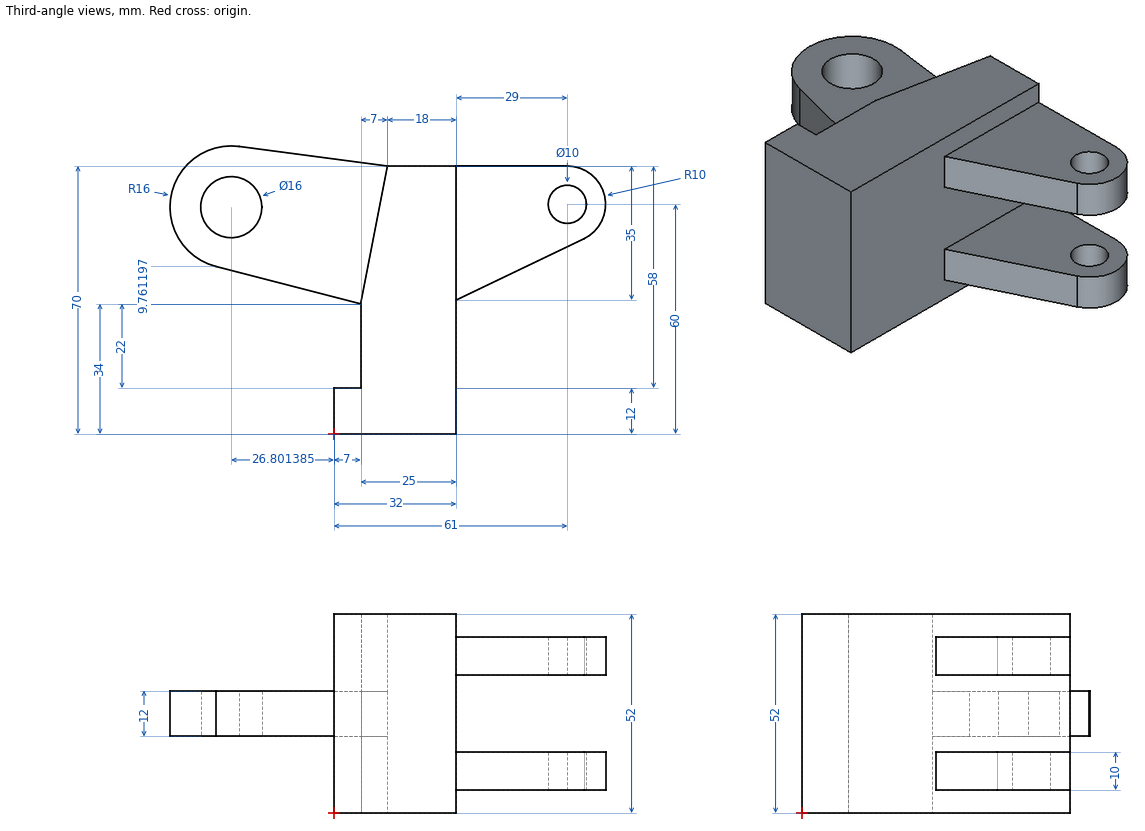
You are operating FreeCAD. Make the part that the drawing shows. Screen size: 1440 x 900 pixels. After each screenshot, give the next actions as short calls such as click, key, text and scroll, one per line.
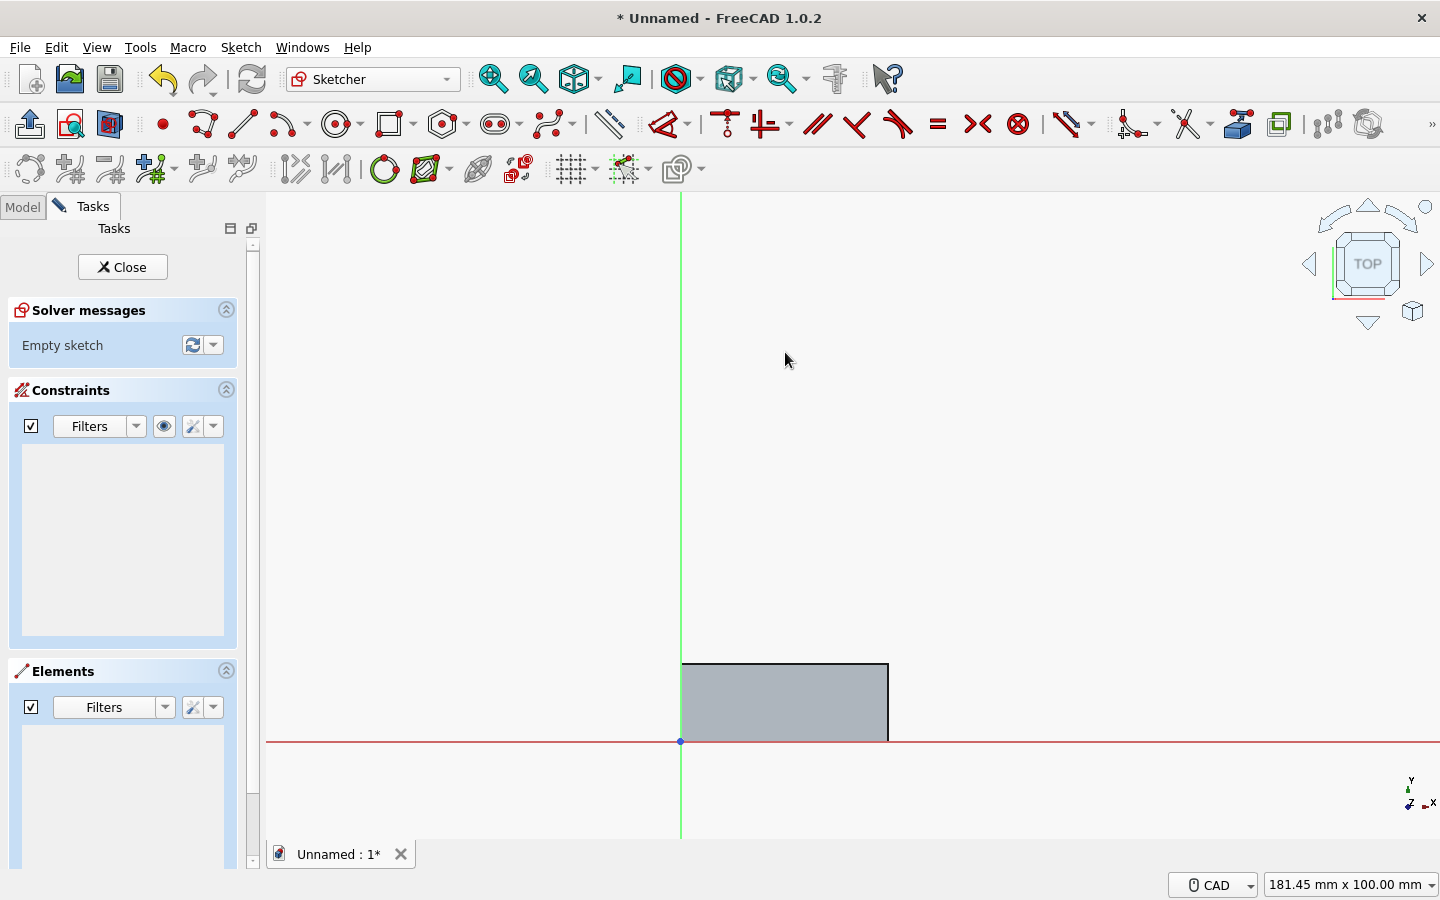
key(g)
key(m)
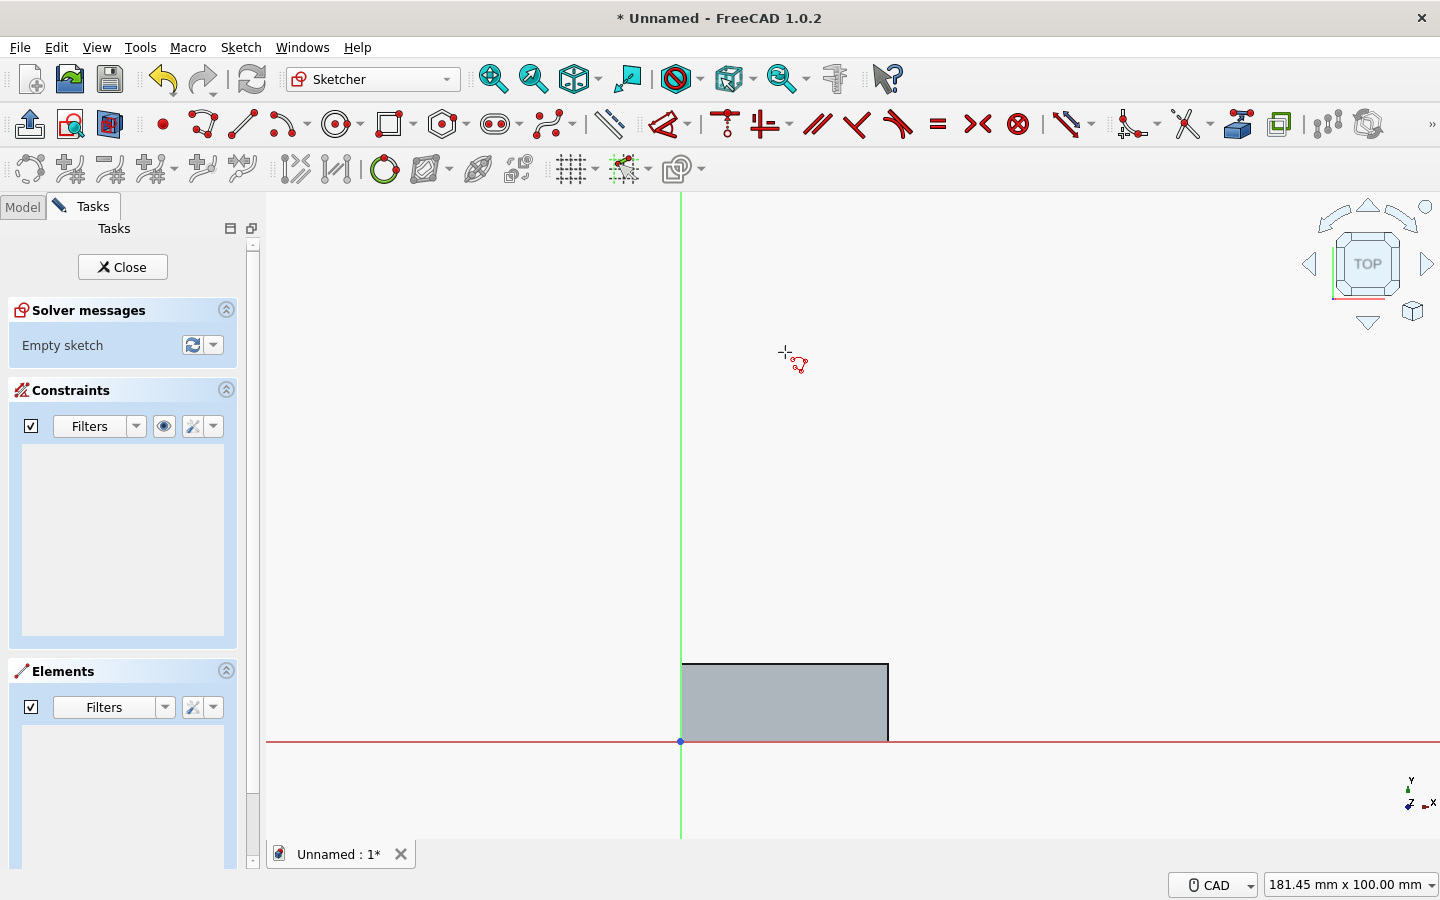
click(726, 664)
click(888, 664)
click(888, 289)
click(771, 289)
click(726, 522)
click(726, 665)
key(Escape)
key(Escape)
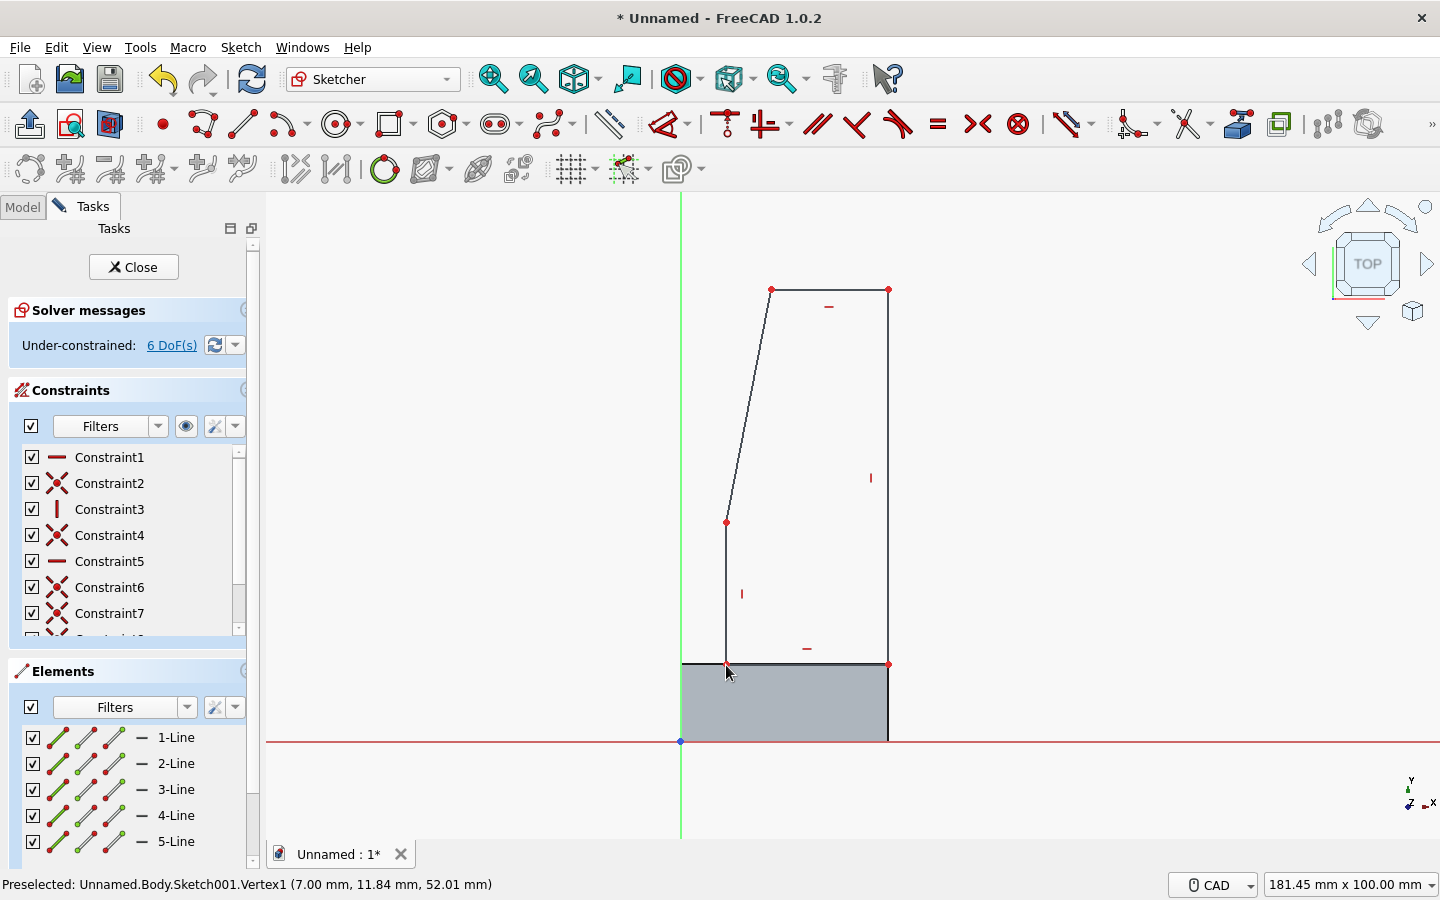
click(664, 124)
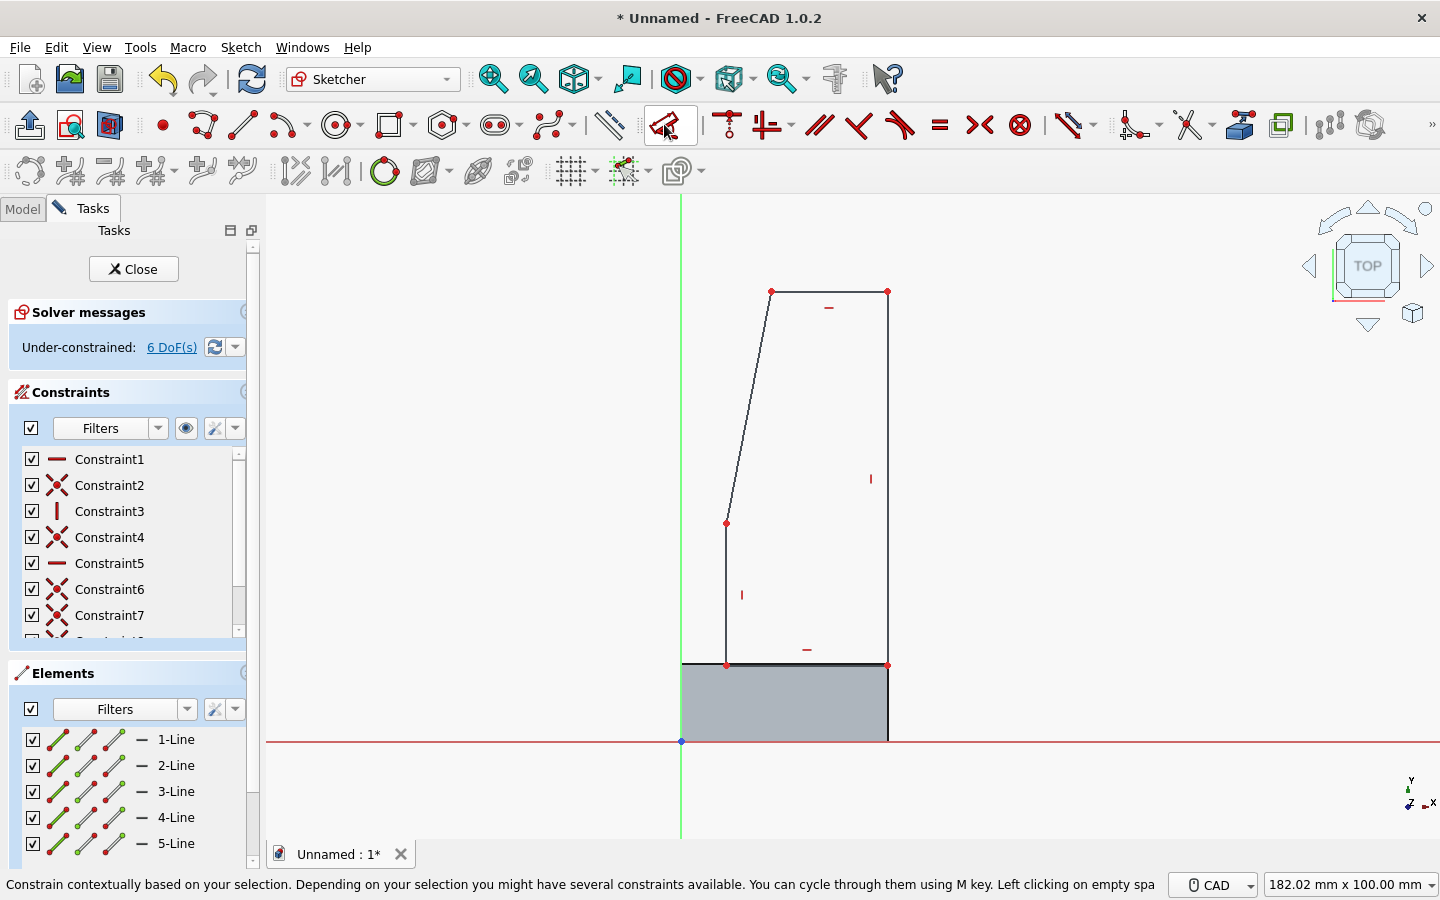
click(775, 666)
click(807, 700)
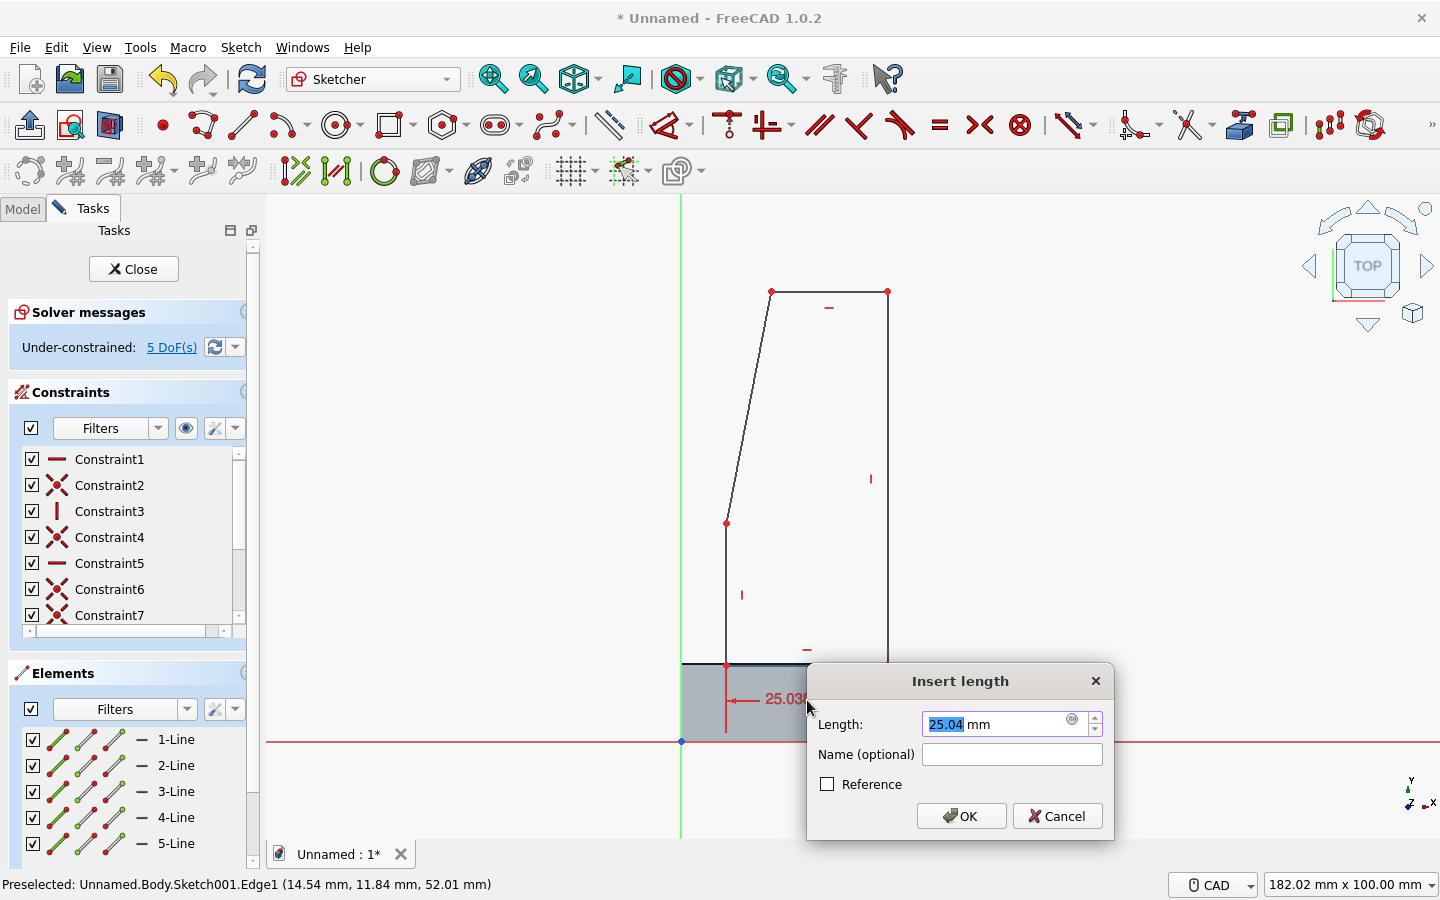
text(25)
key(Return)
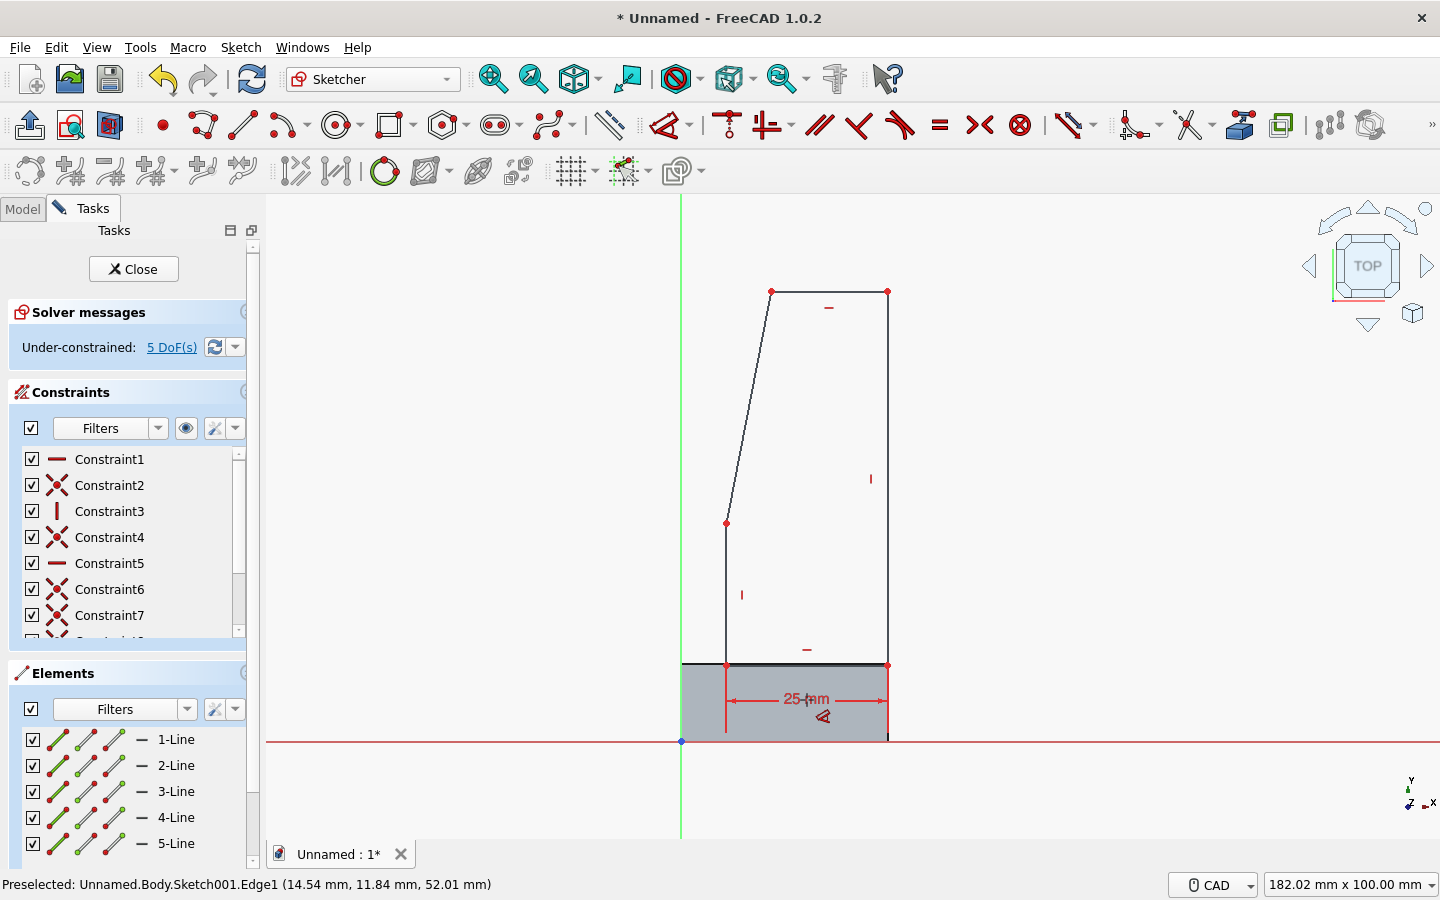
click(888, 553)
click(922, 479)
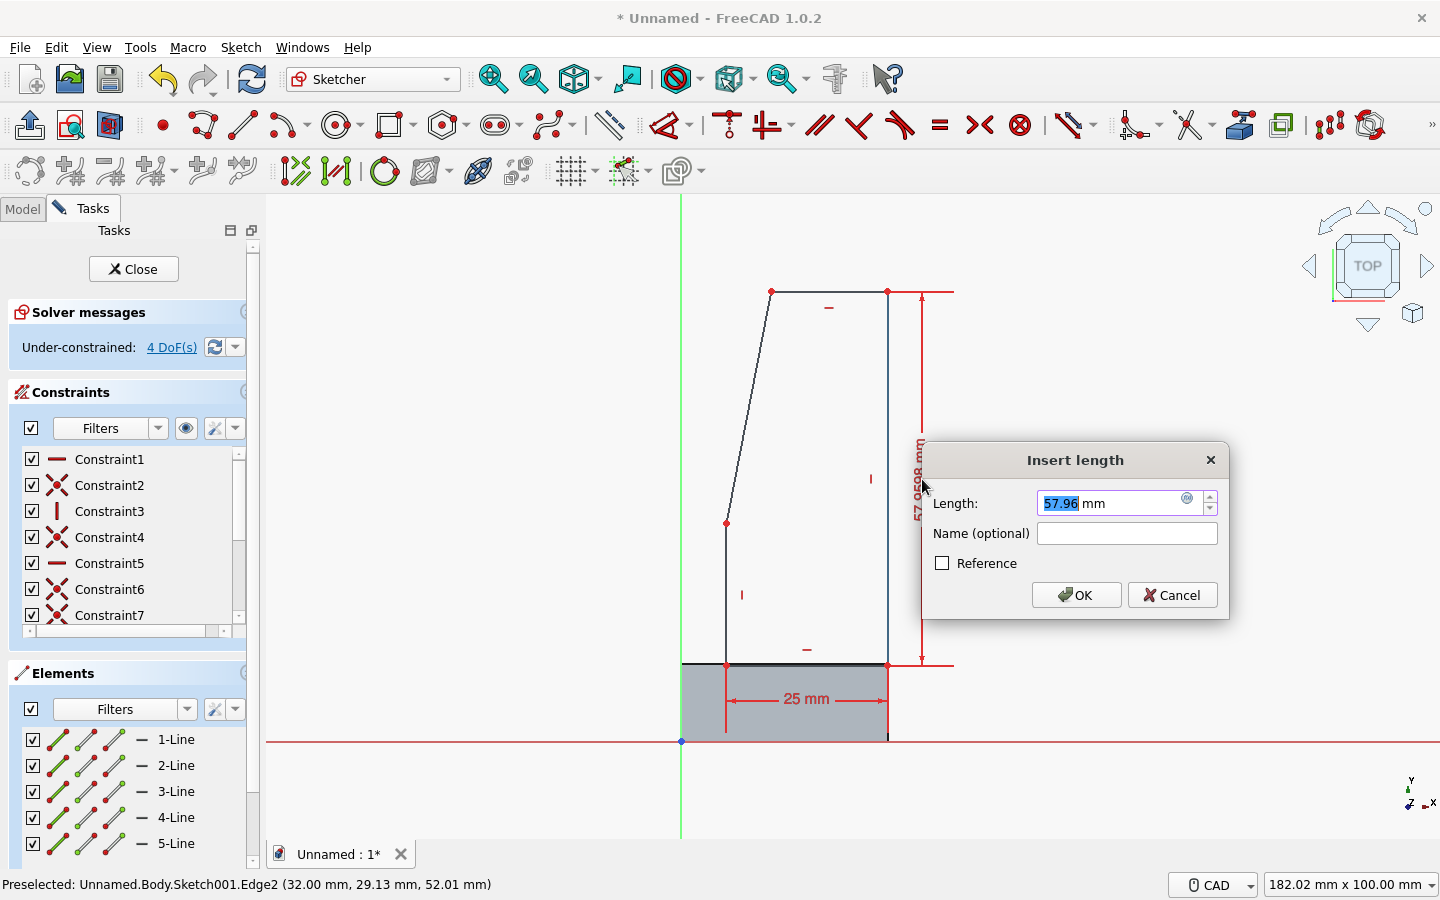
text(58)
key(Return)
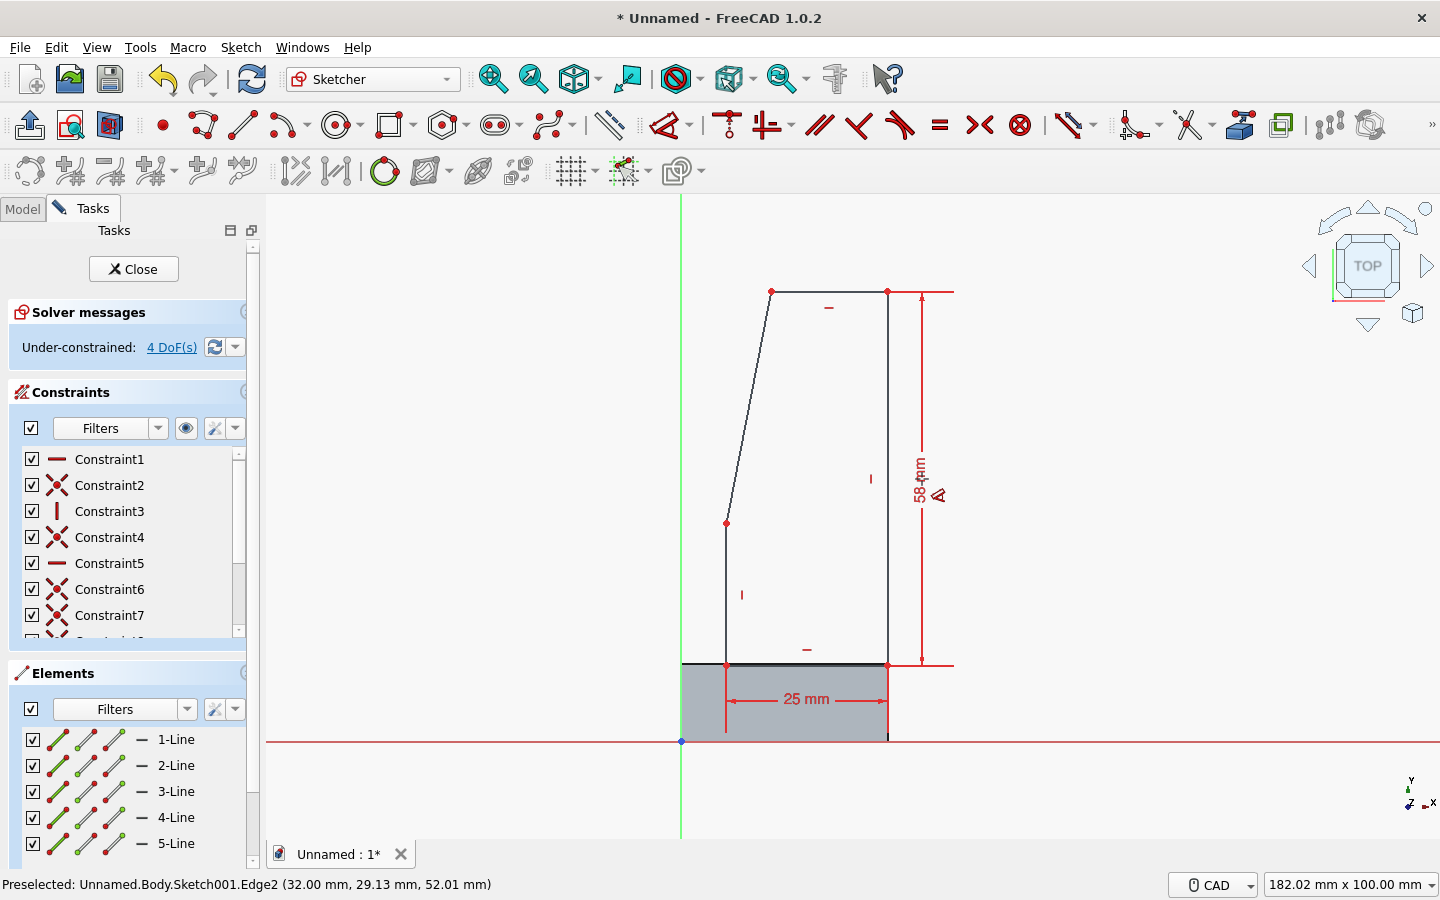
click(853, 292)
click(829, 258)